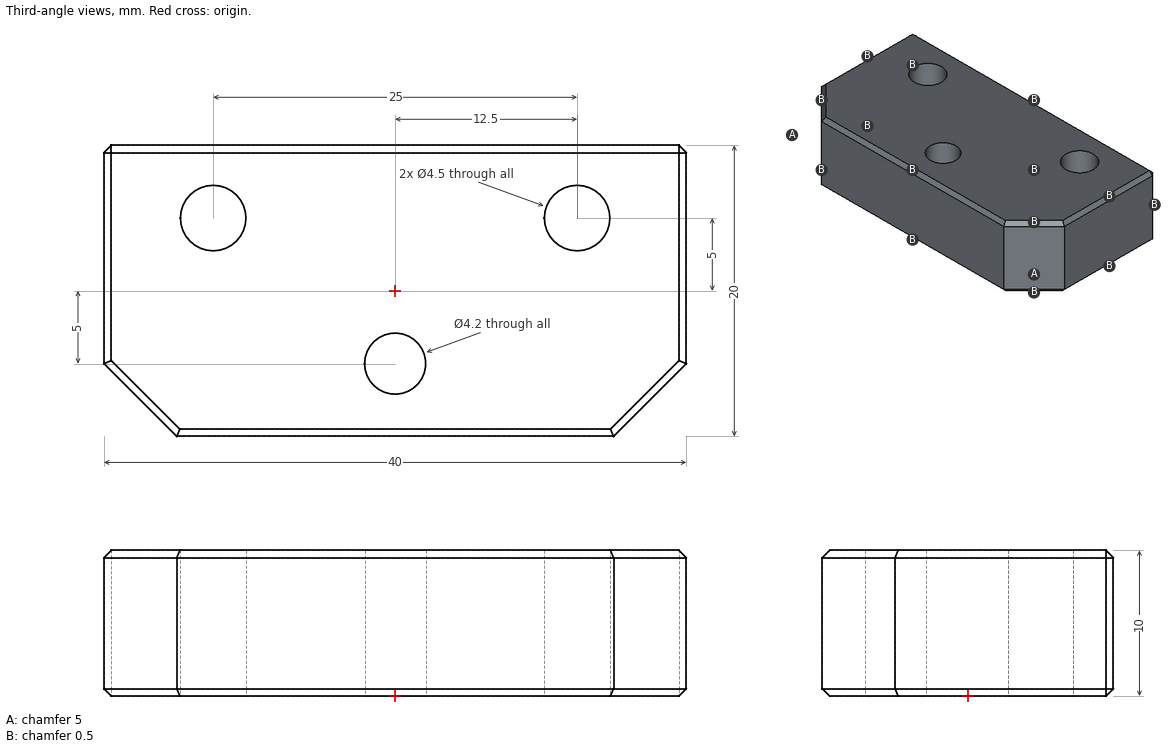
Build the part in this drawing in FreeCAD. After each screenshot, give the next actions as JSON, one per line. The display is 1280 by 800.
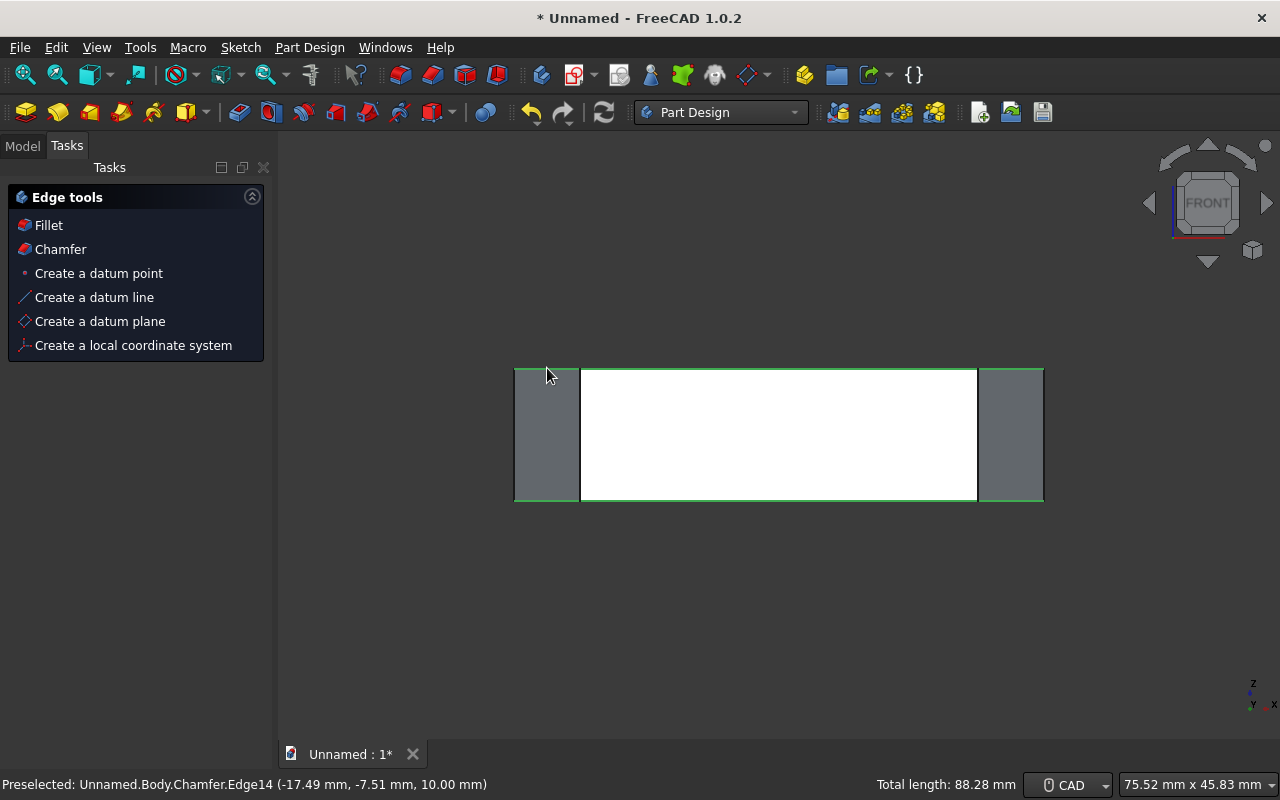
{"action": "key", "text": "0"}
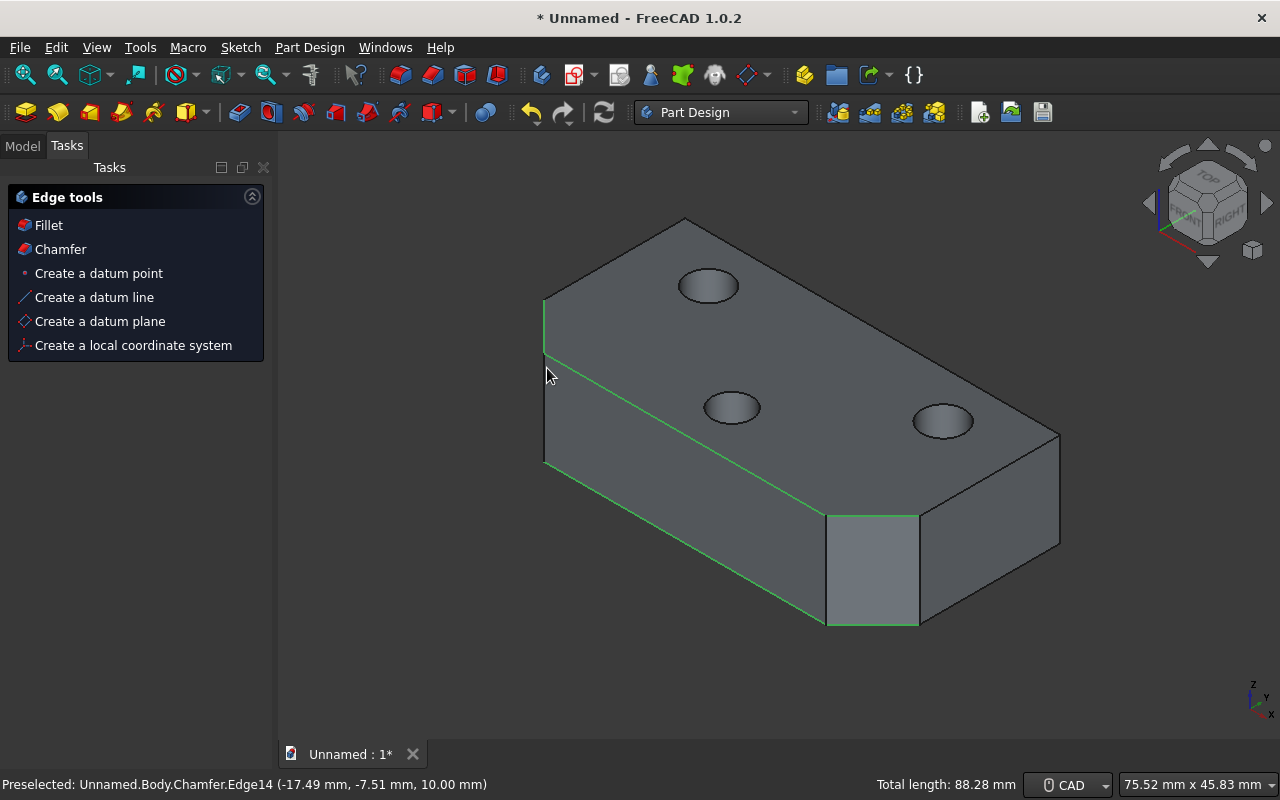
{"action": "left_click", "coordinate": [990, 475], "text": "ctrl"}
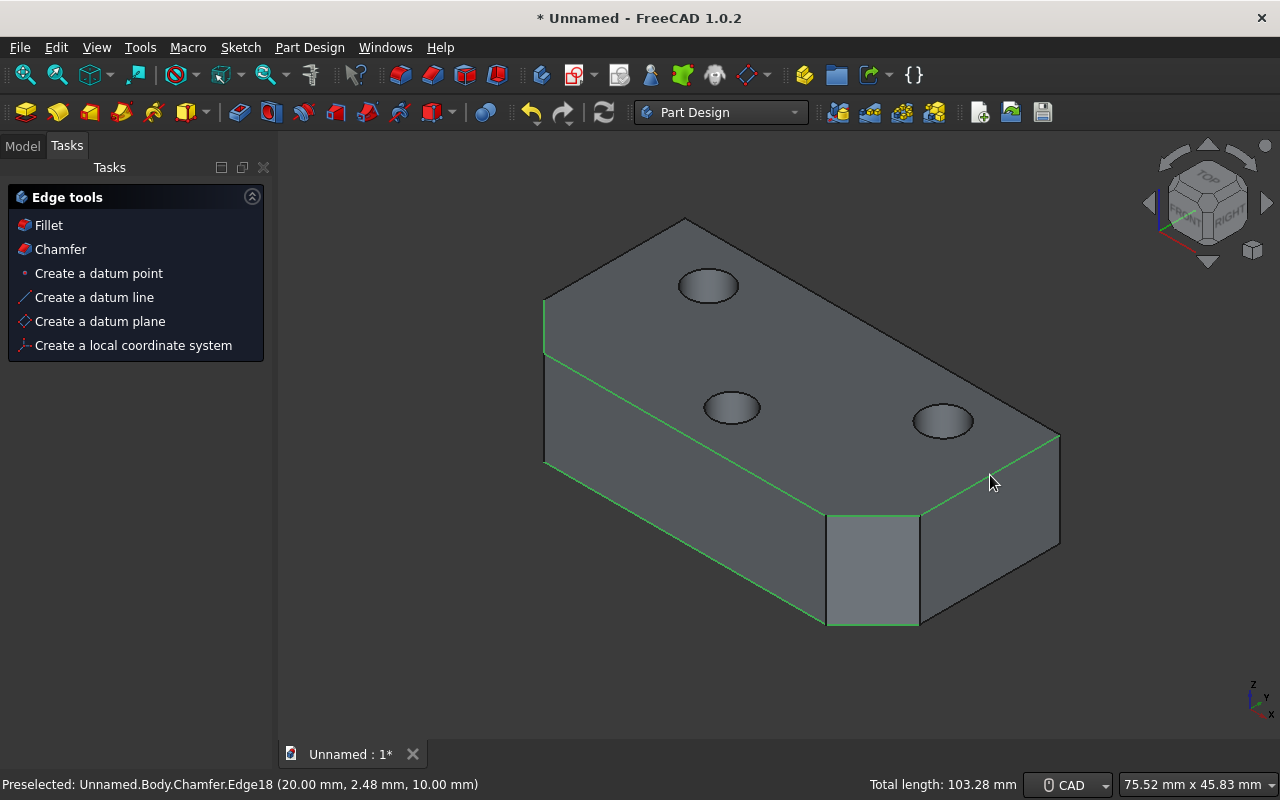
{"action": "key", "text": "2"}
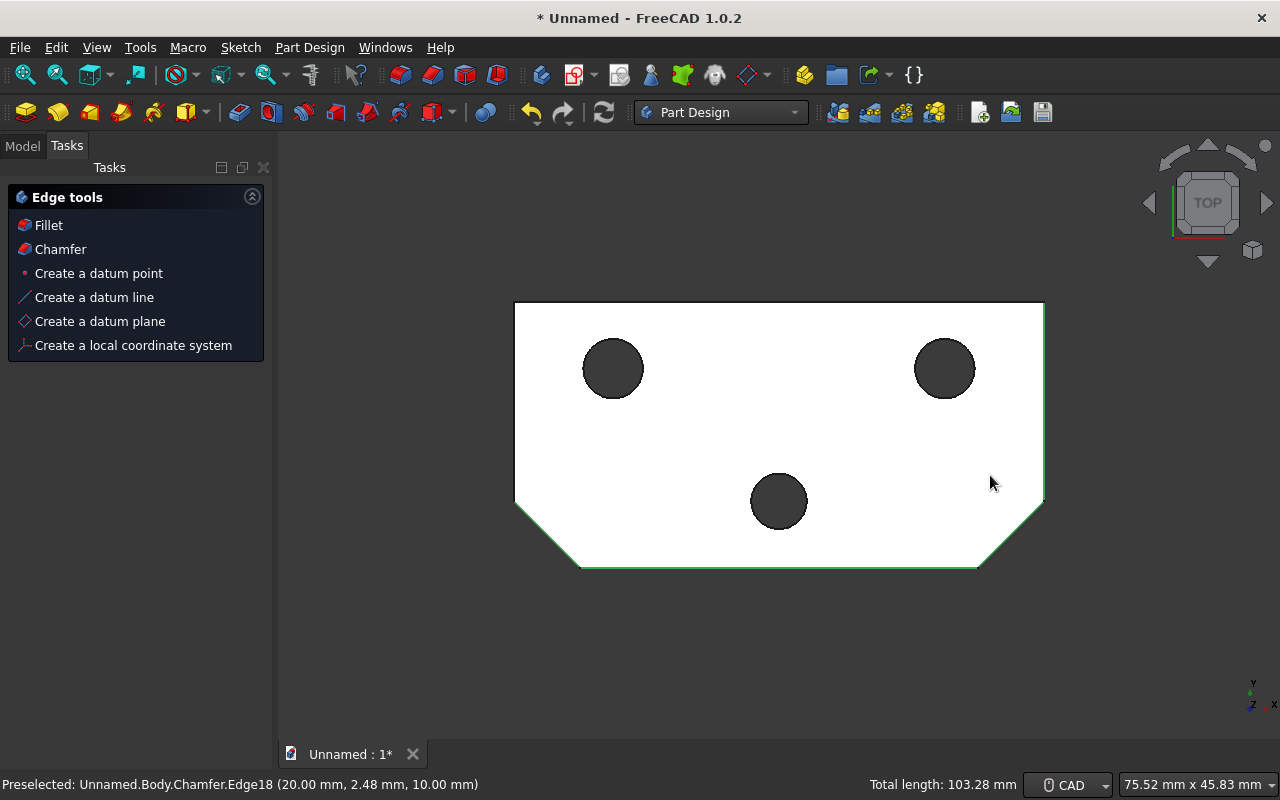
{"action": "left_click", "coordinate": [514, 401], "text": "ctrl"}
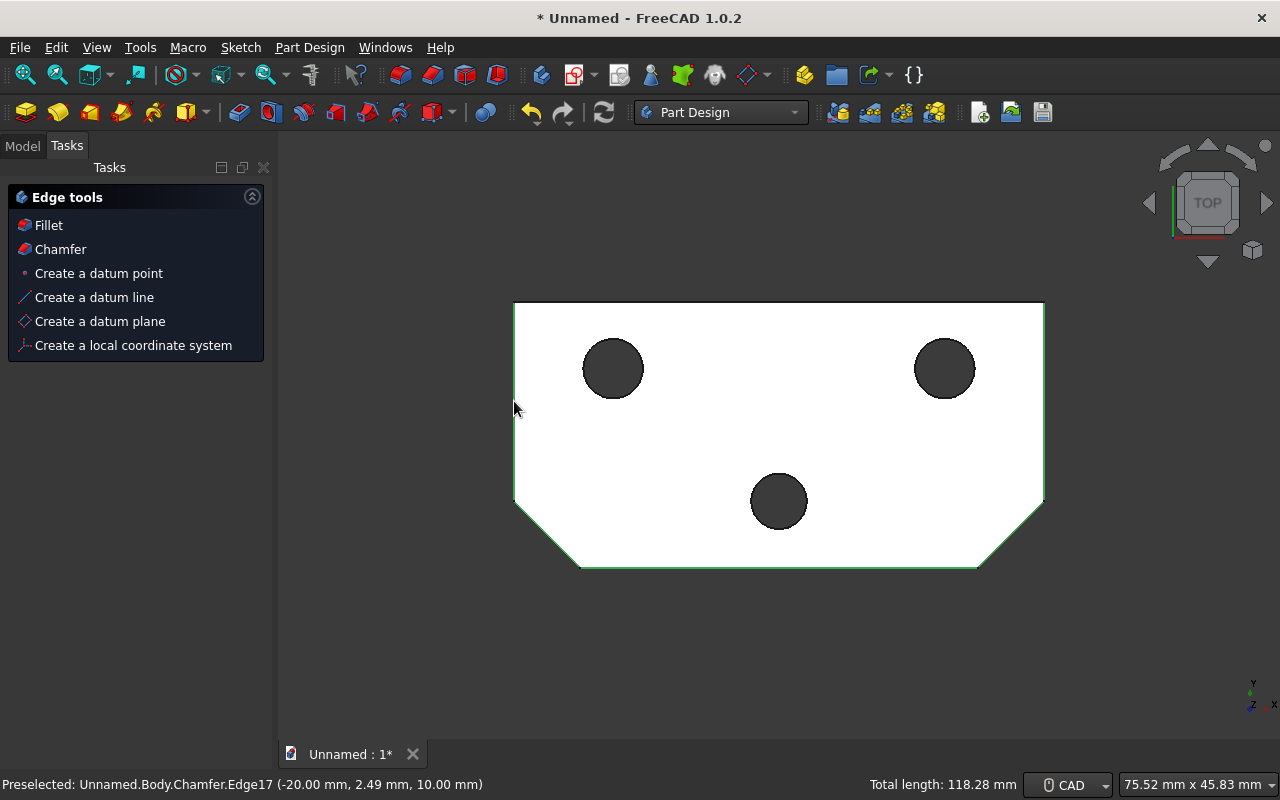
{"action": "key", "text": "1"}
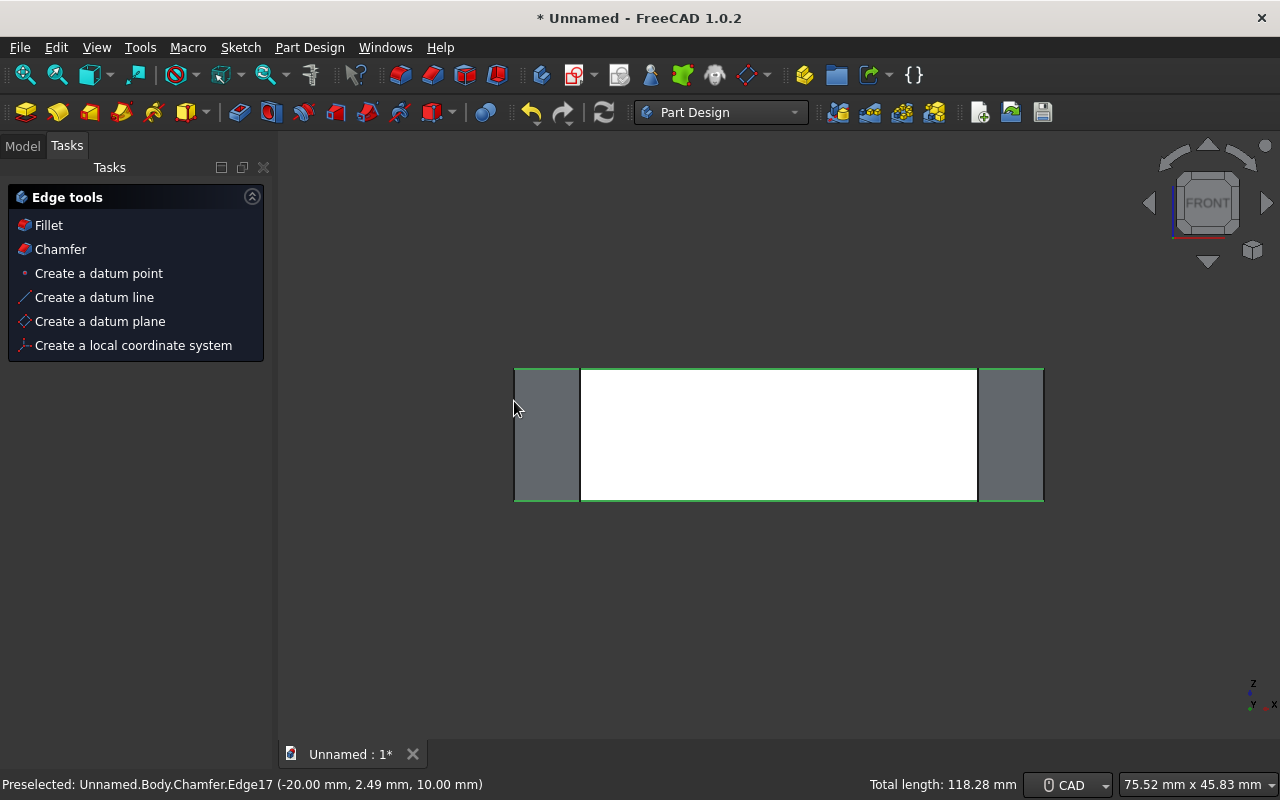
{"action": "key", "text": "3"}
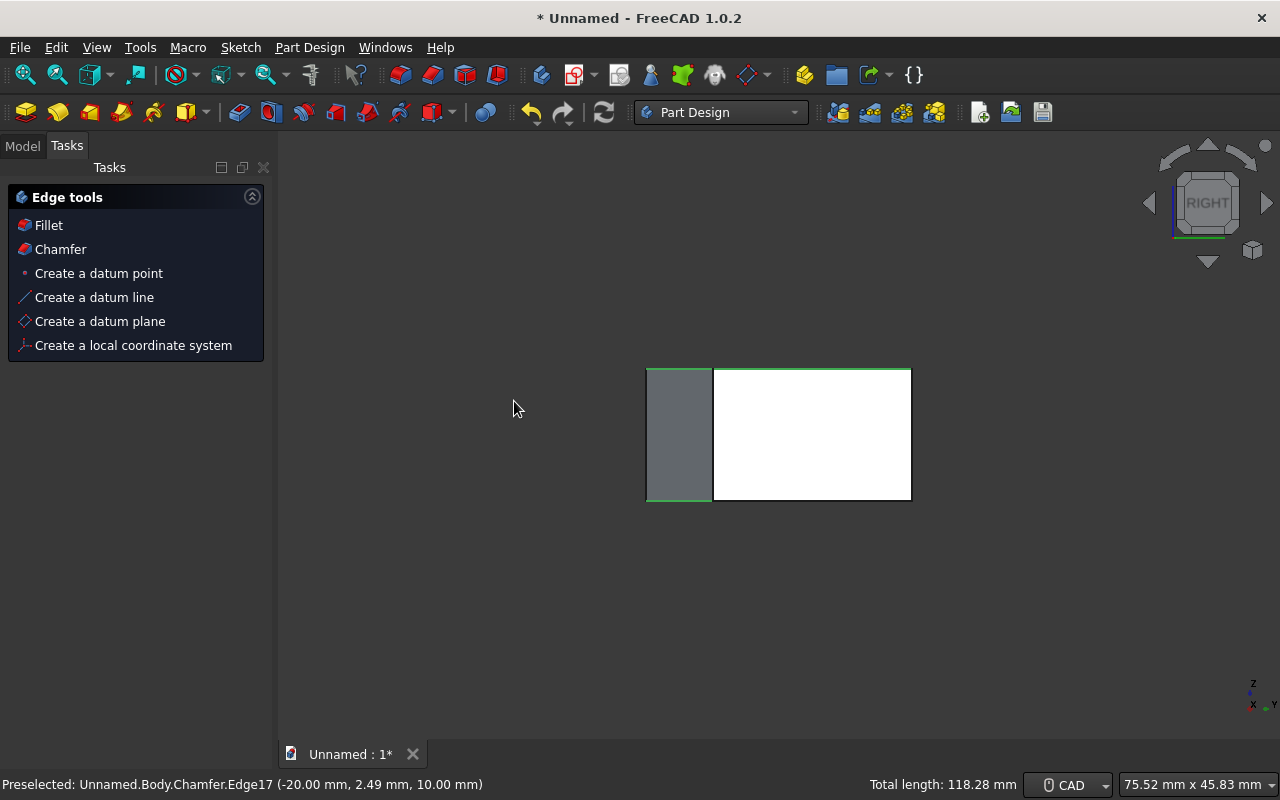
{"action": "left_click", "coordinate": [26, 76]}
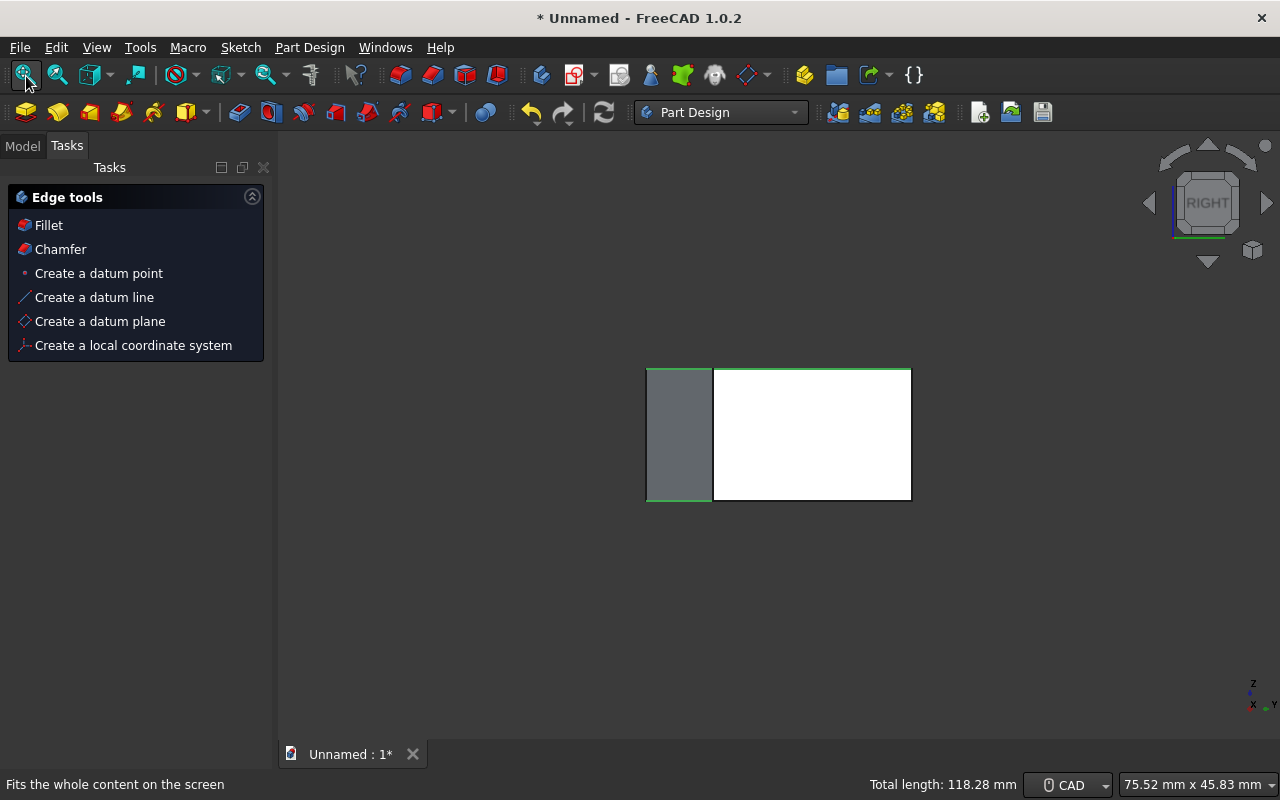
{"action": "left_click", "coordinate": [812, 500], "text": "ctrl"}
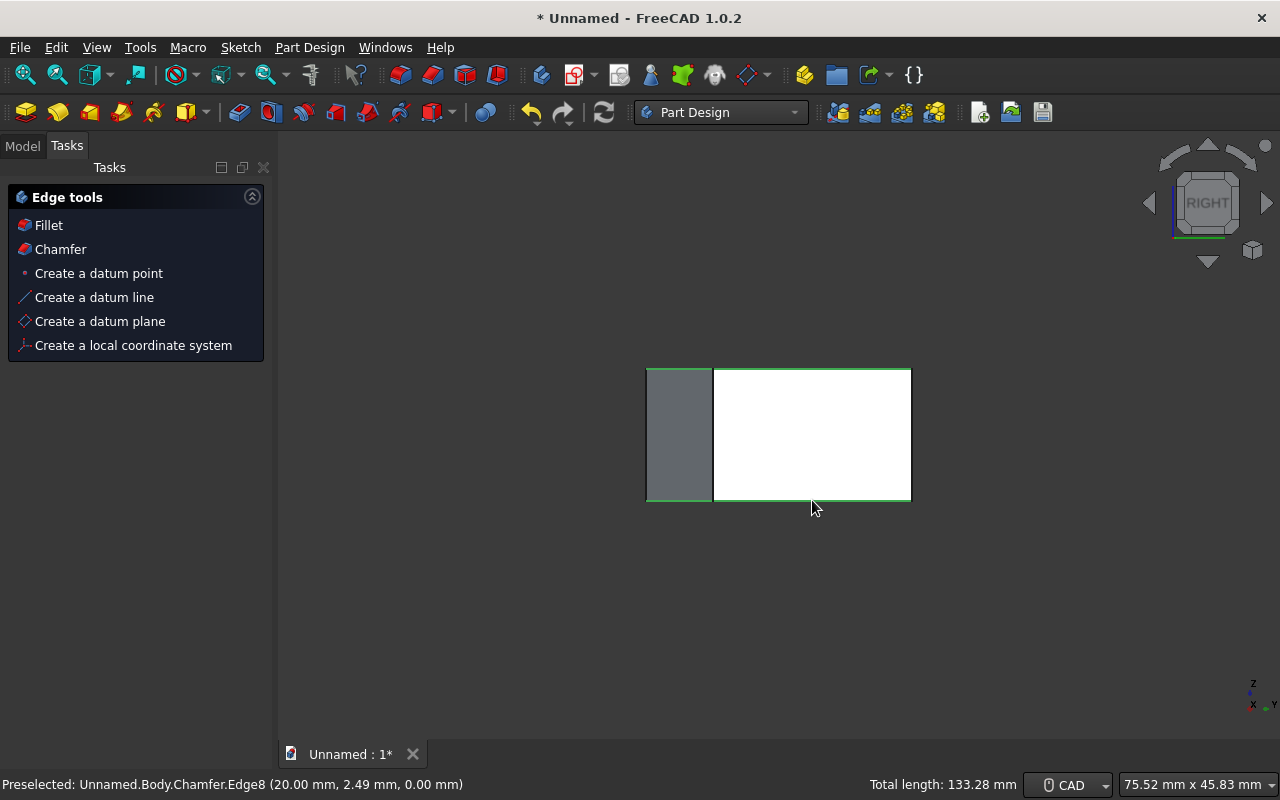
{"action": "key", "text": "5"}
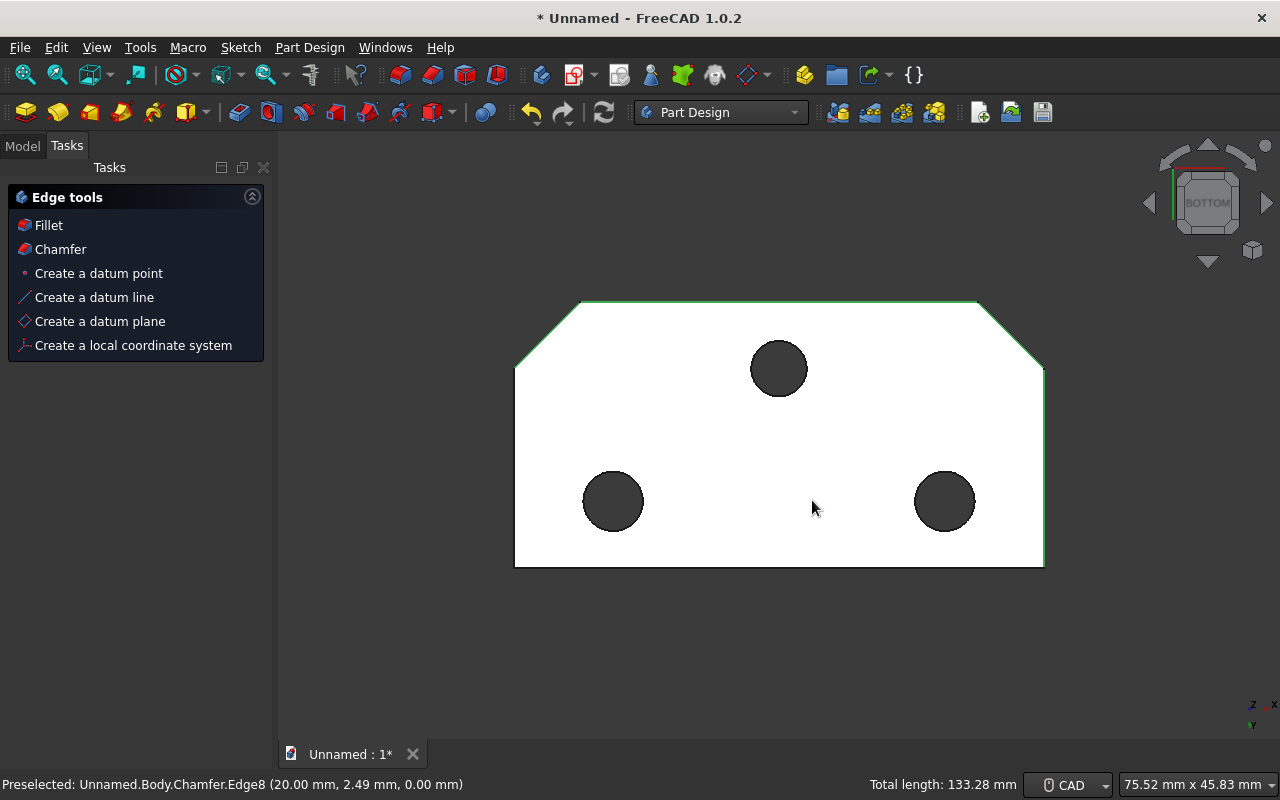
{"action": "left_click", "coordinate": [514, 467], "text": "ctrl"}